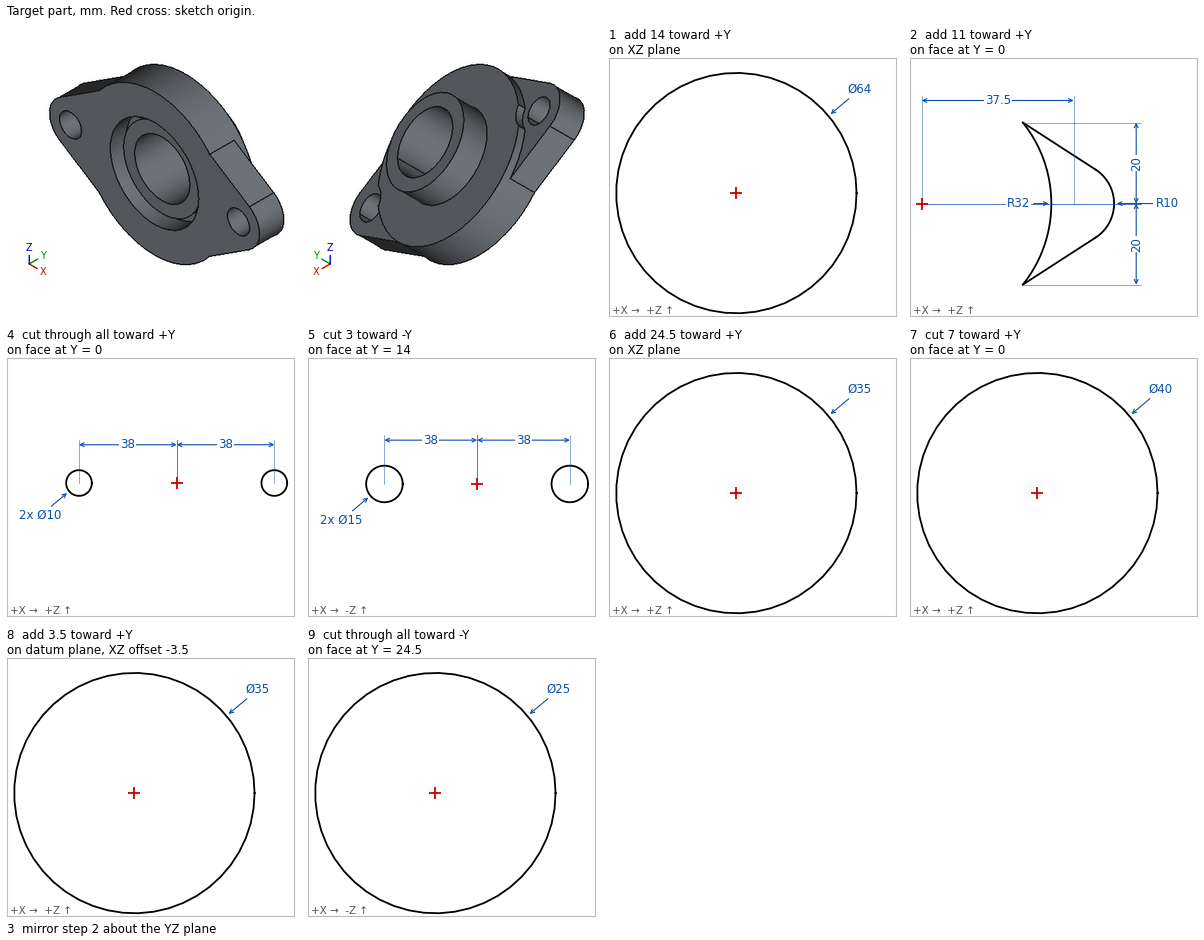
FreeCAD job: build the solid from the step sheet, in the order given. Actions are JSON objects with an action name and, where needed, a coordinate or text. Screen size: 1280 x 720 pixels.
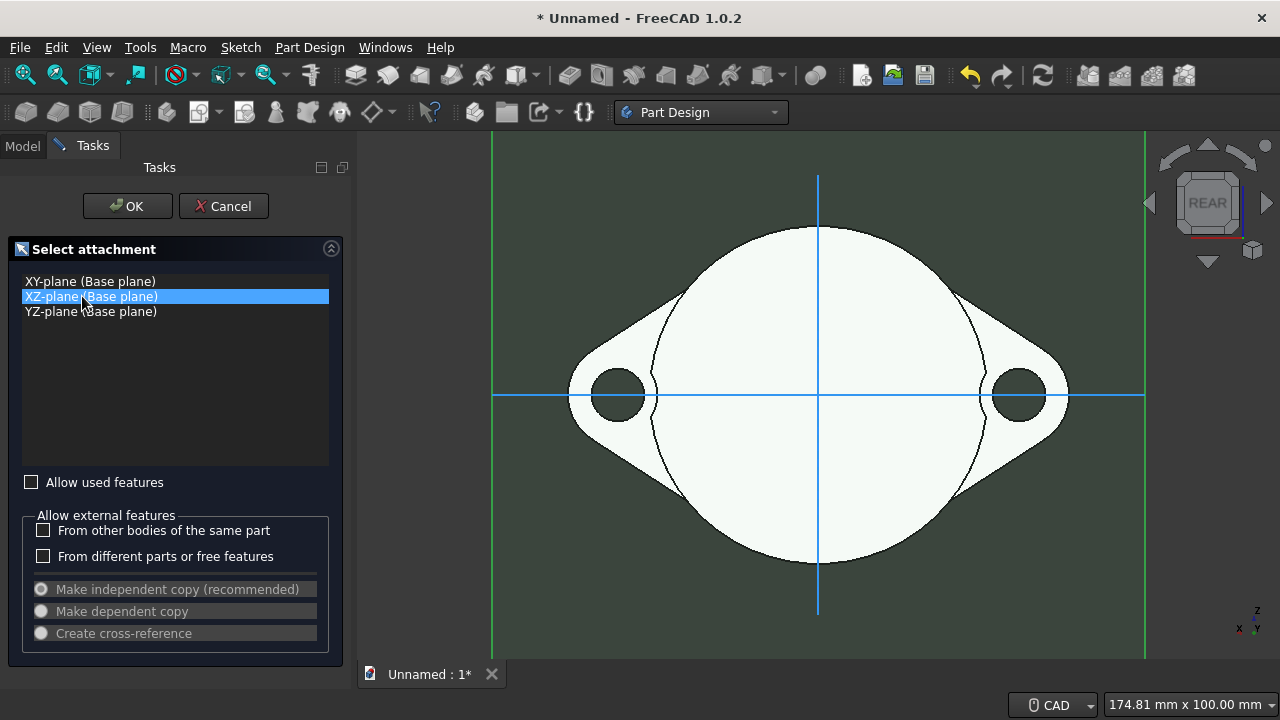
{"action": "left_click", "coordinate": [128, 206]}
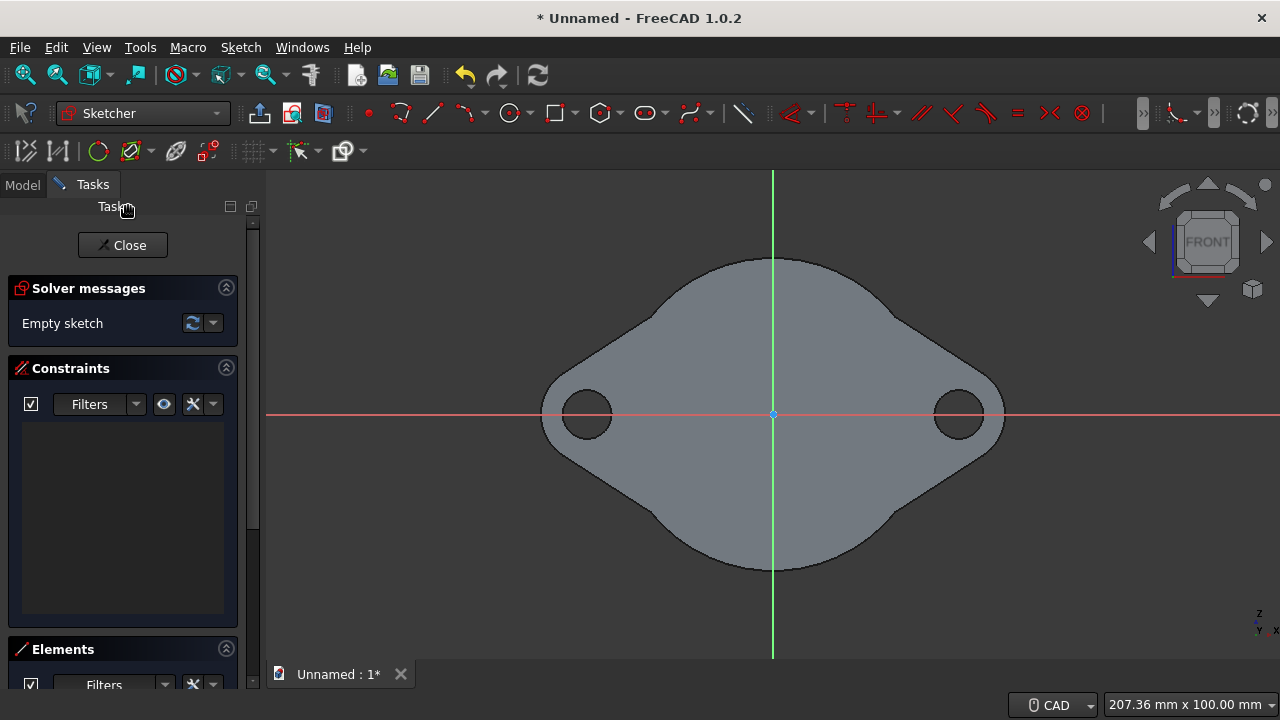
{"action": "scroll", "coordinate": [856, 415], "scroll_direction": "up", "scroll_amount": 3}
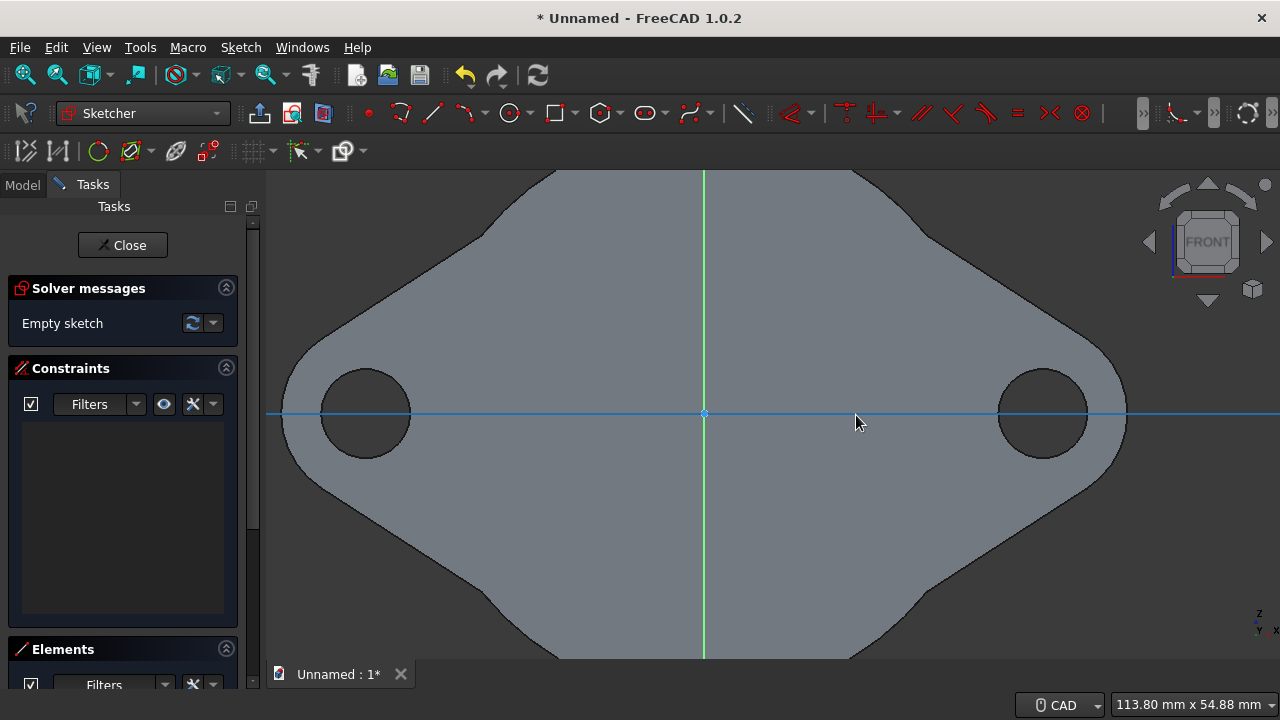
{"action": "key", "text": "g c"}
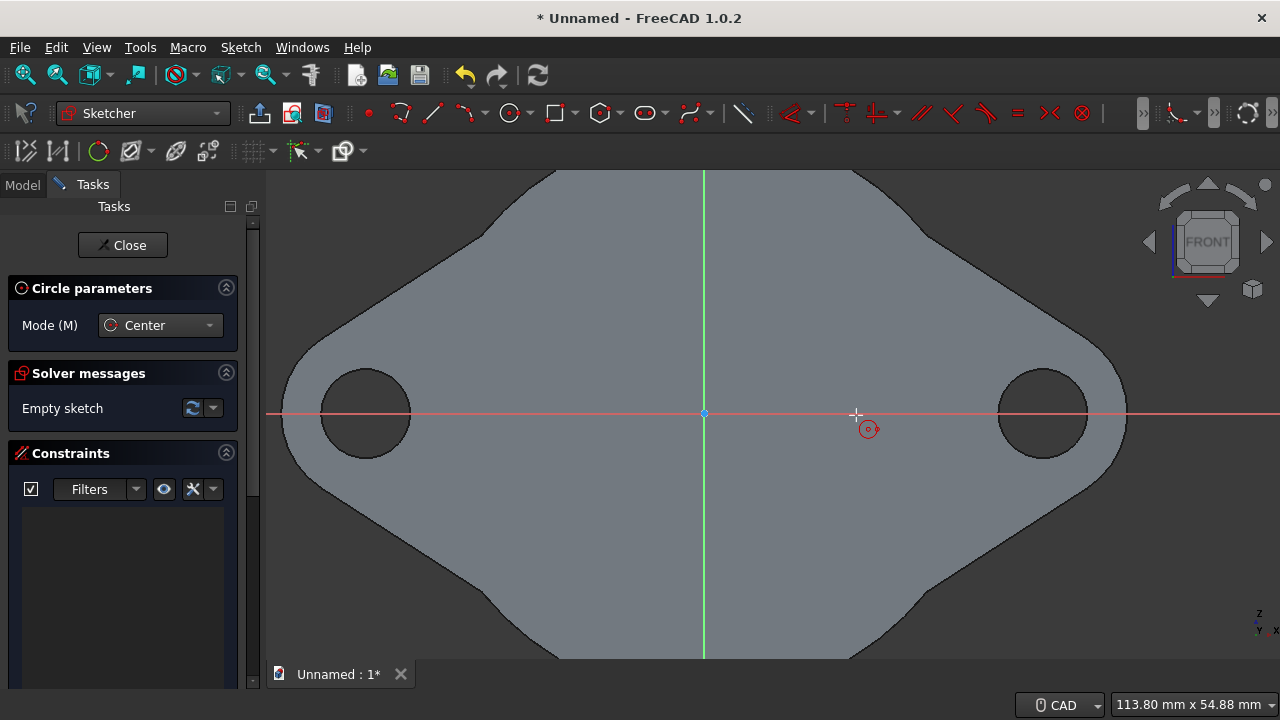
{"action": "left_click", "coordinate": [704, 414]}
{"action": "left_click", "coordinate": [815, 303]}
{"action": "key", "text": "Escape"}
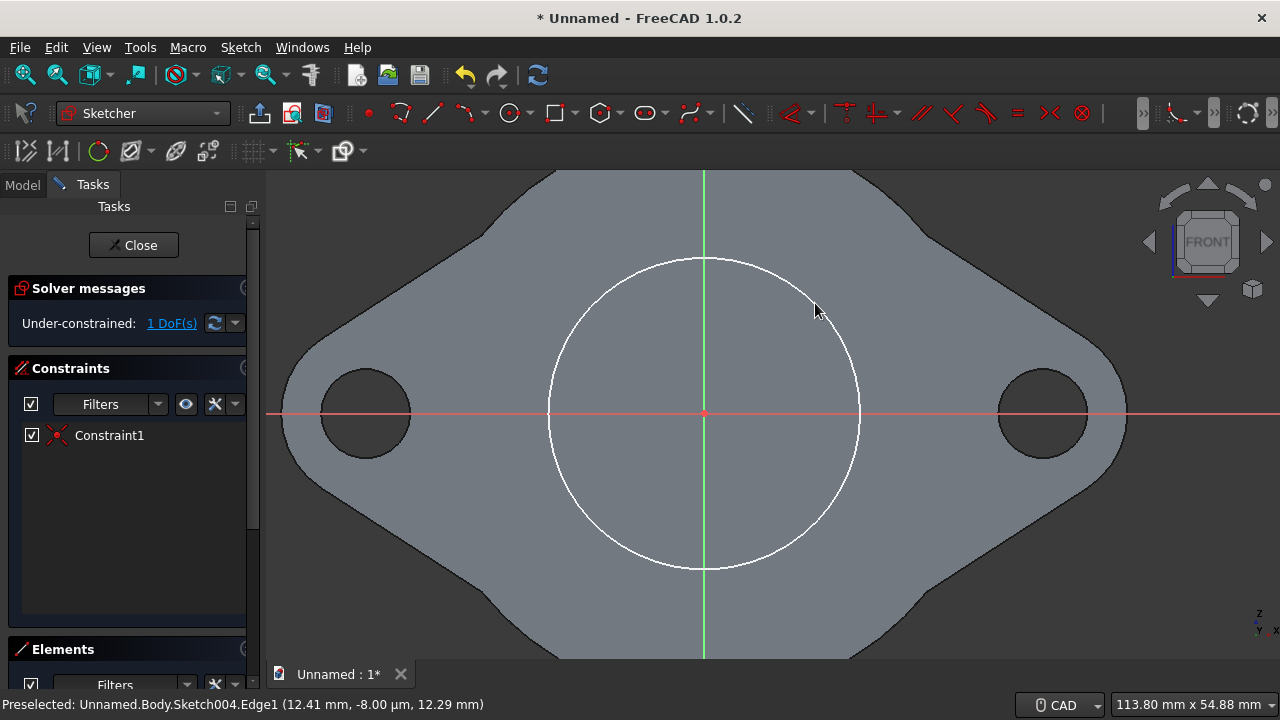
{"action": "left_click", "coordinate": [790, 114]}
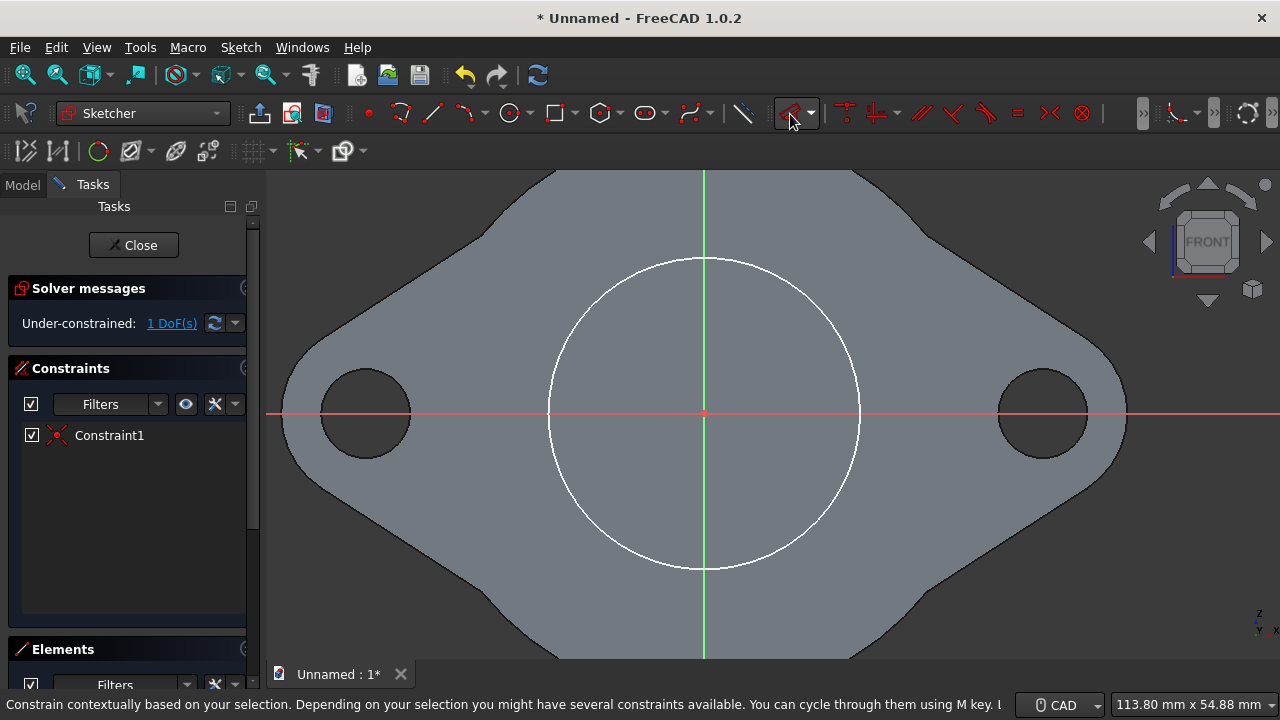
{"action": "left_click", "coordinate": [814, 303]}
{"action": "left_click", "coordinate": [837, 280]}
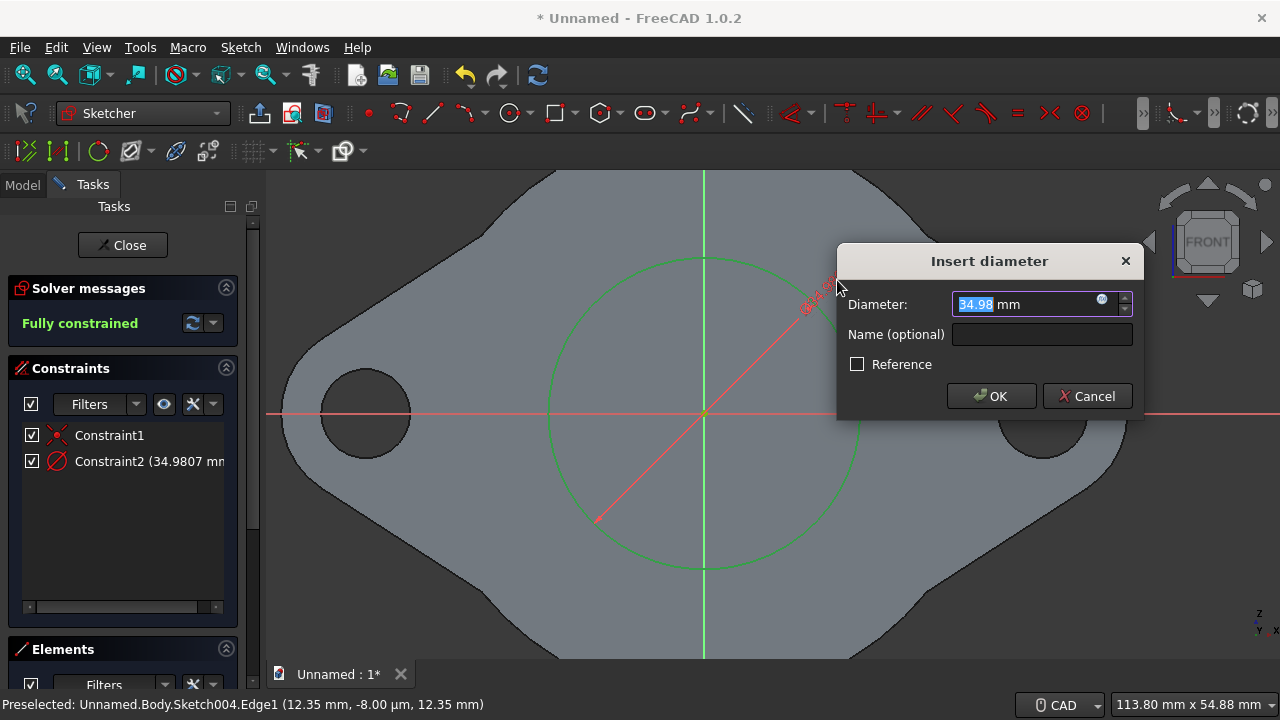
{"action": "type", "text": "35"}
{"action": "key", "text": "Return"}
{"action": "key", "text": "Escape"}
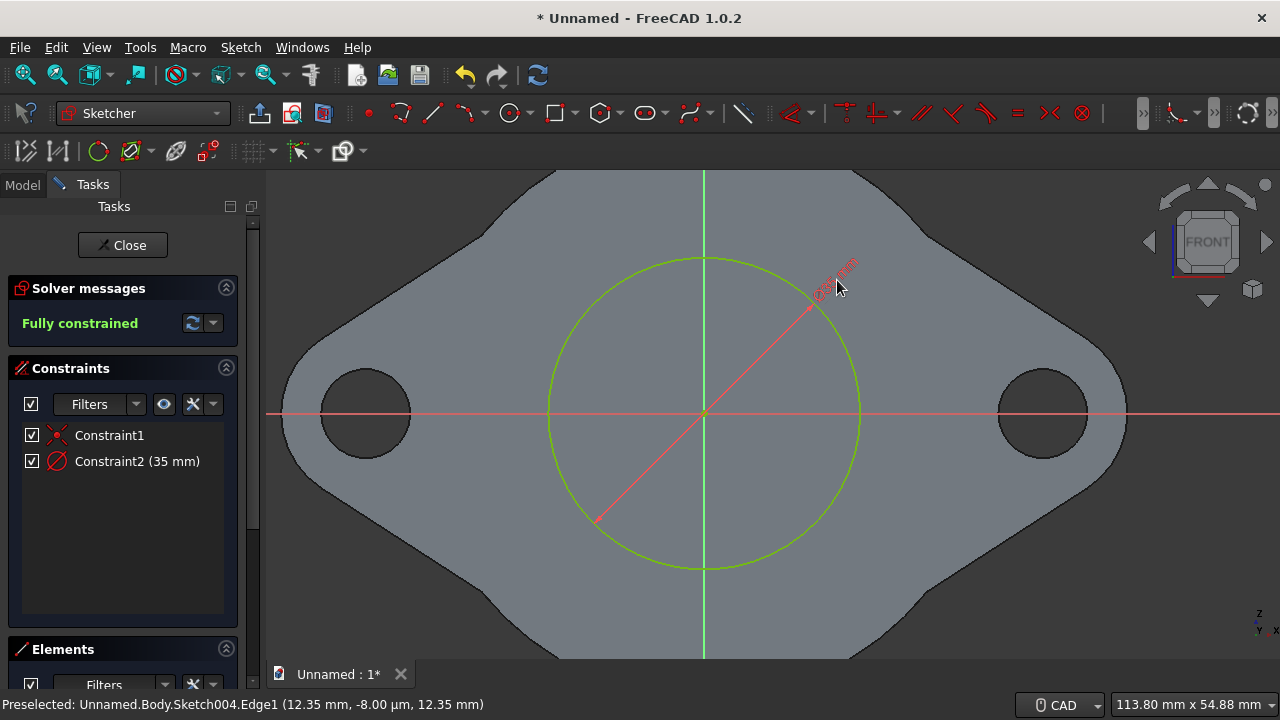
{"action": "left_click", "coordinate": [123, 245]}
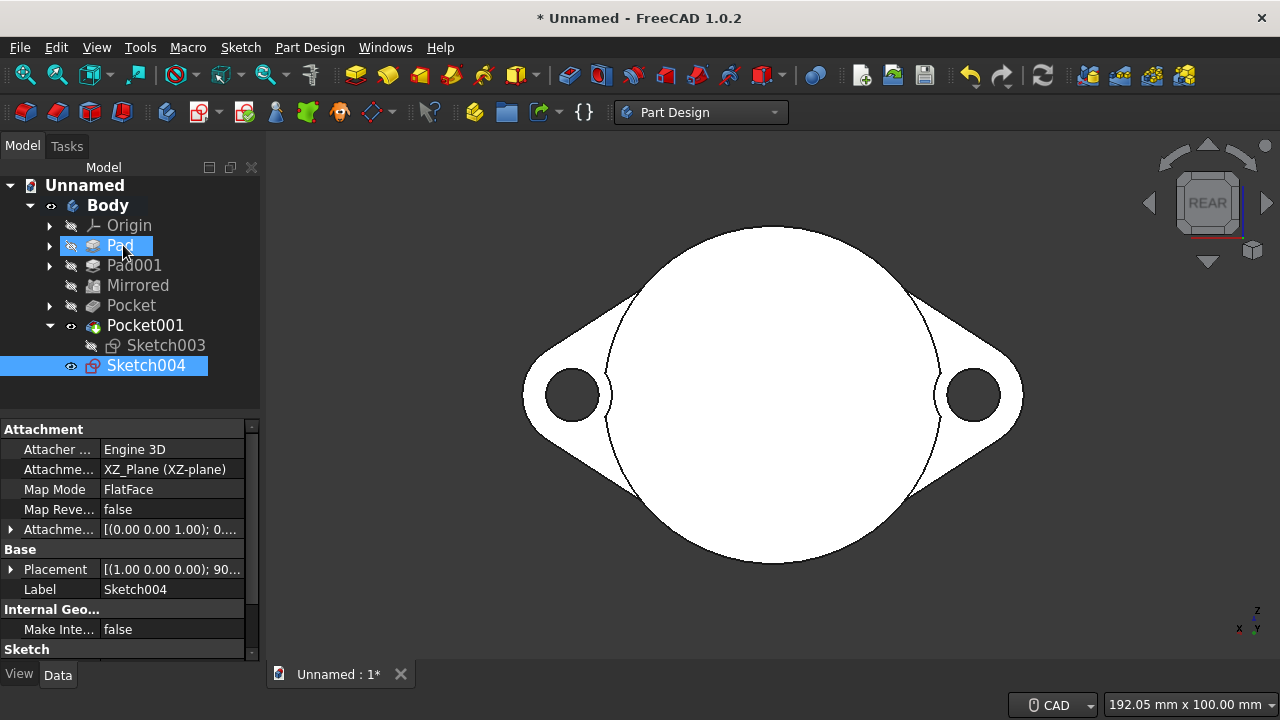
{"action": "left_click", "coordinate": [356, 76]}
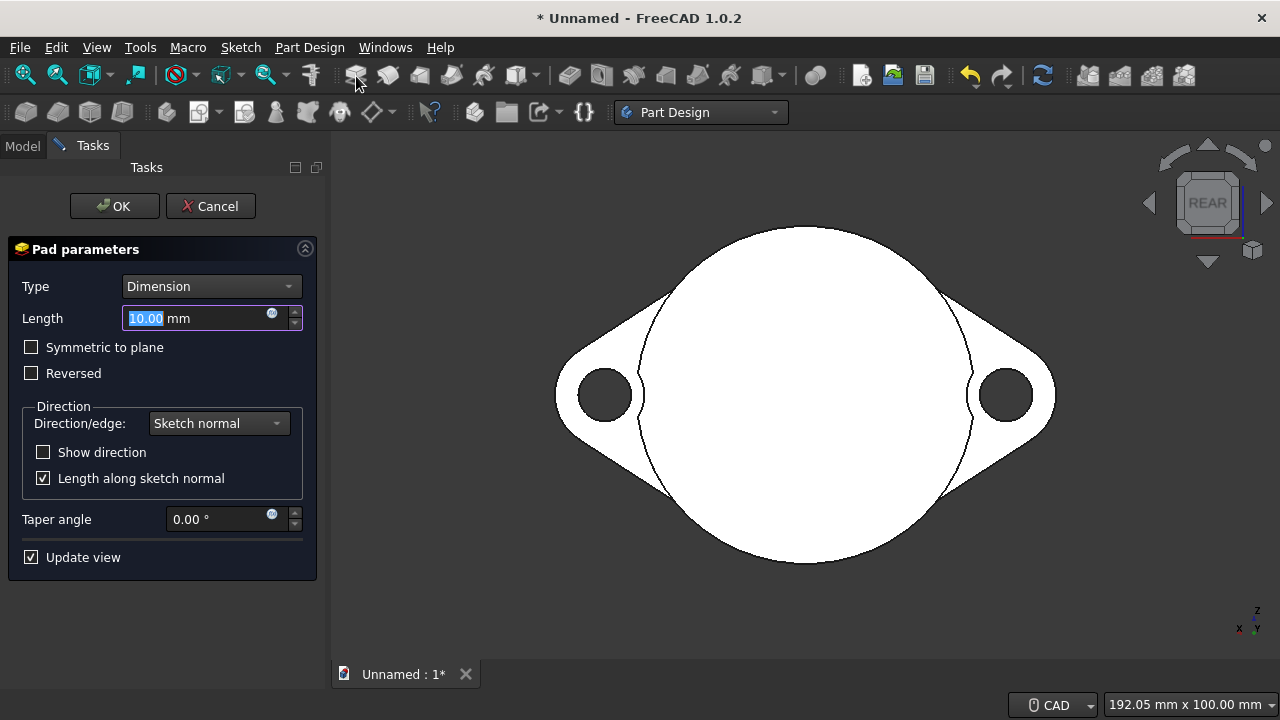
{"action": "type", "text": "24.5"}
{"action": "key", "text": "Tab"}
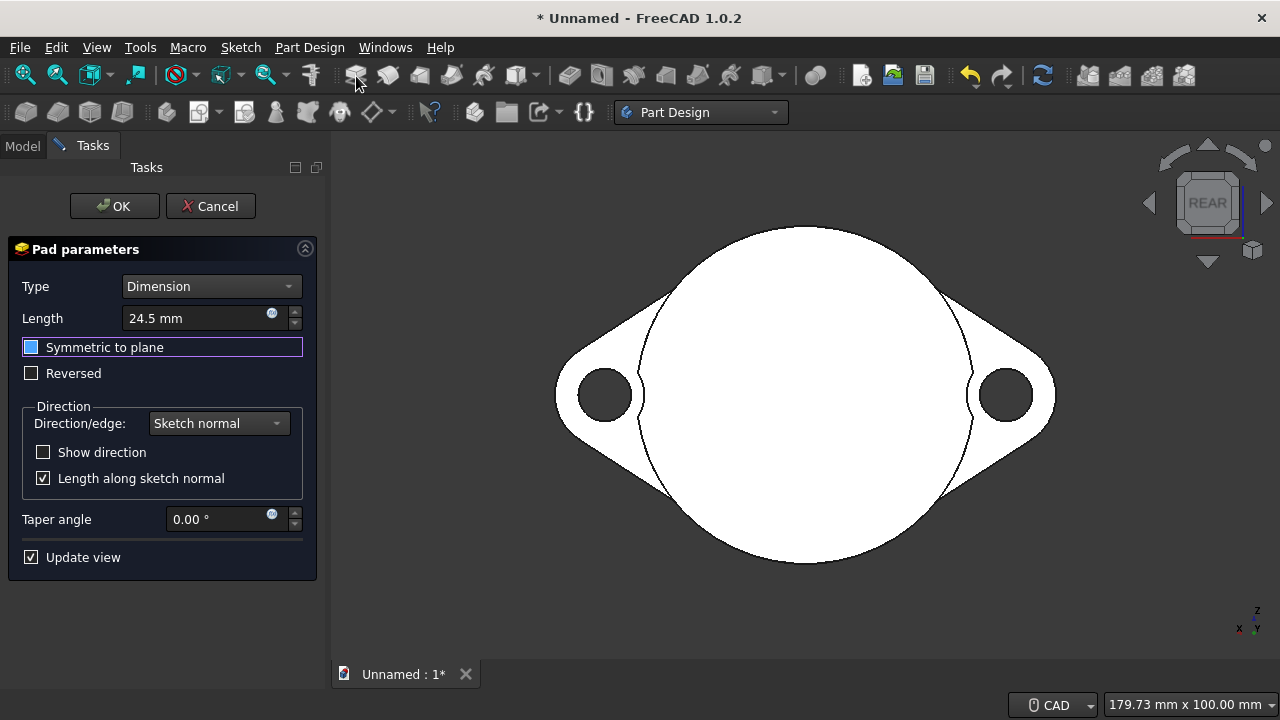
{"action": "left_click", "coordinate": [30, 373]}